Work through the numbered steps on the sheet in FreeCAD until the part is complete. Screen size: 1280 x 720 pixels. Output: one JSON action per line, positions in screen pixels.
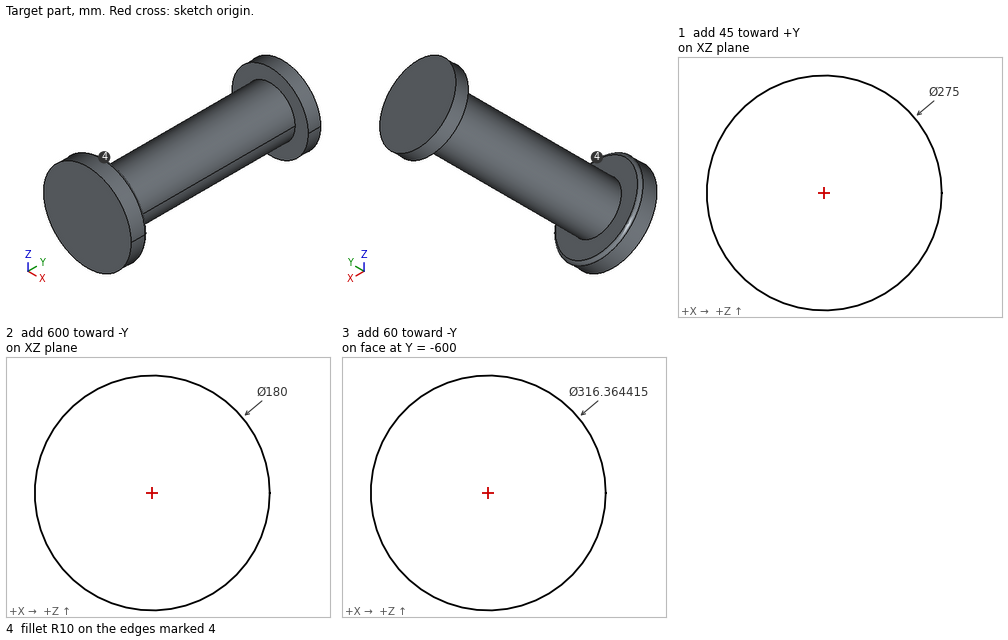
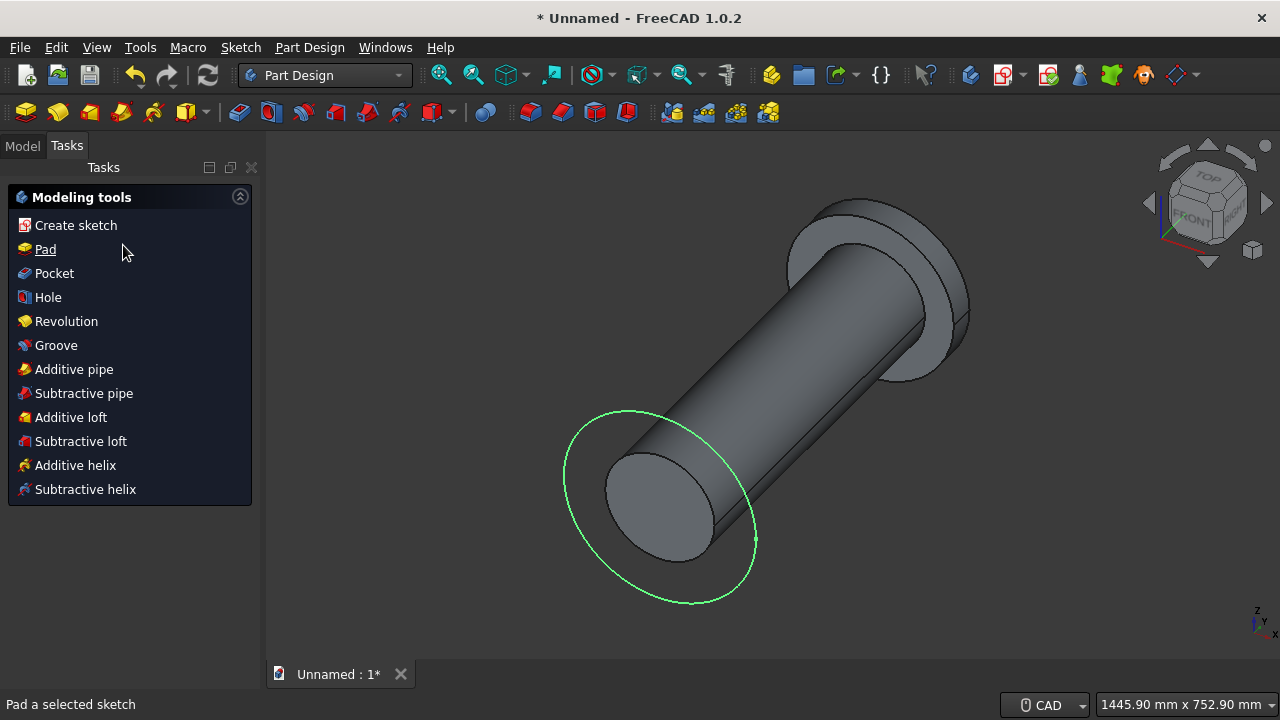
{"action": "left_click", "coordinate": [26, 112]}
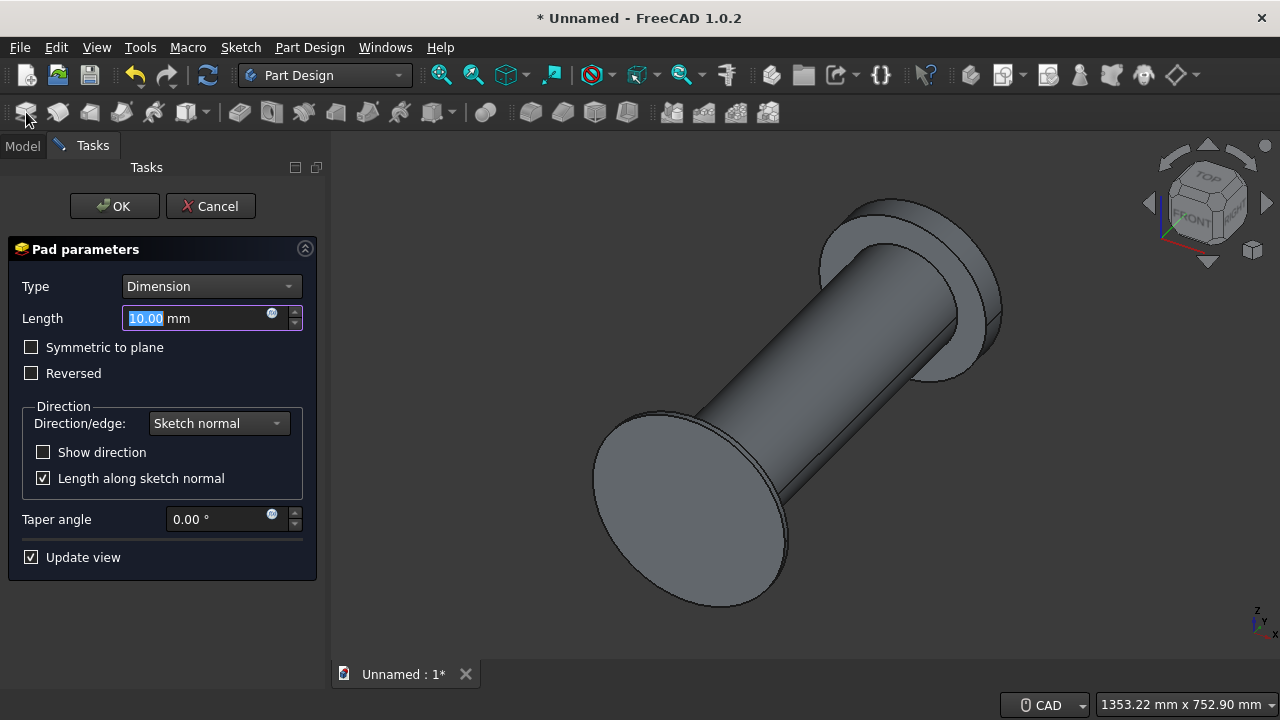
{"action": "type", "text": "60"}
{"action": "key", "text": "Tab"}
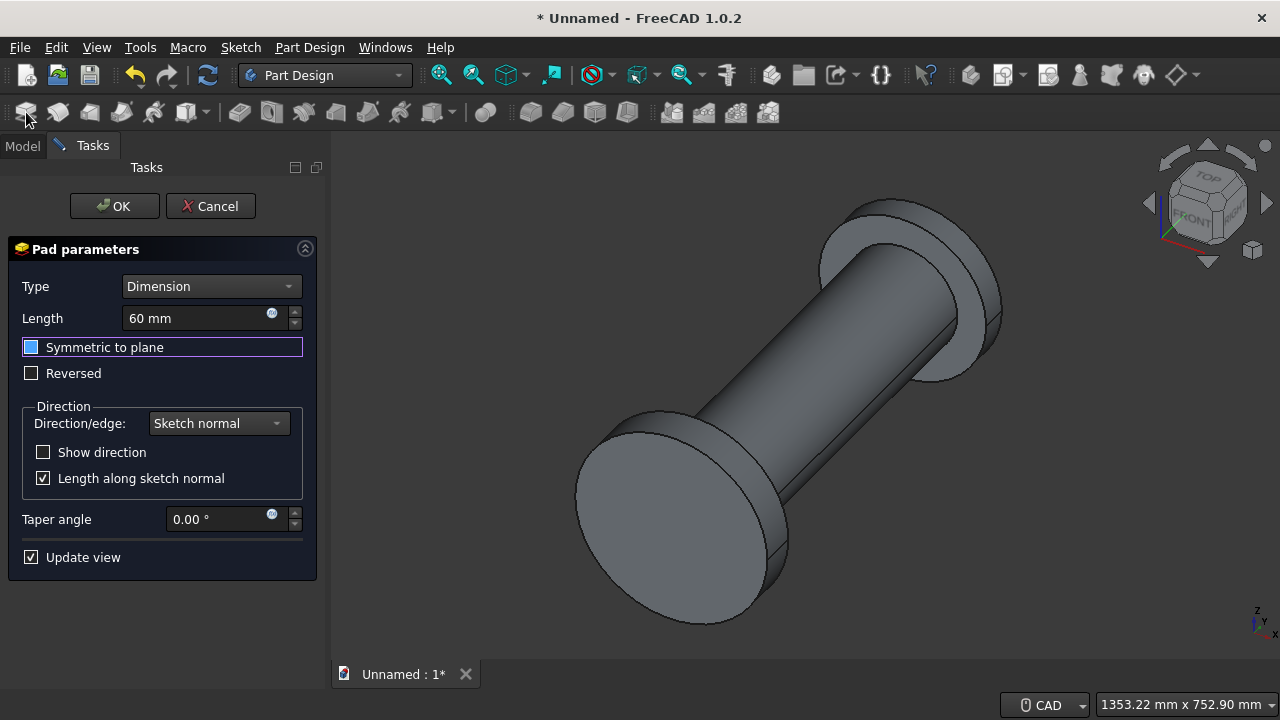
{"action": "left_click", "coordinate": [115, 206]}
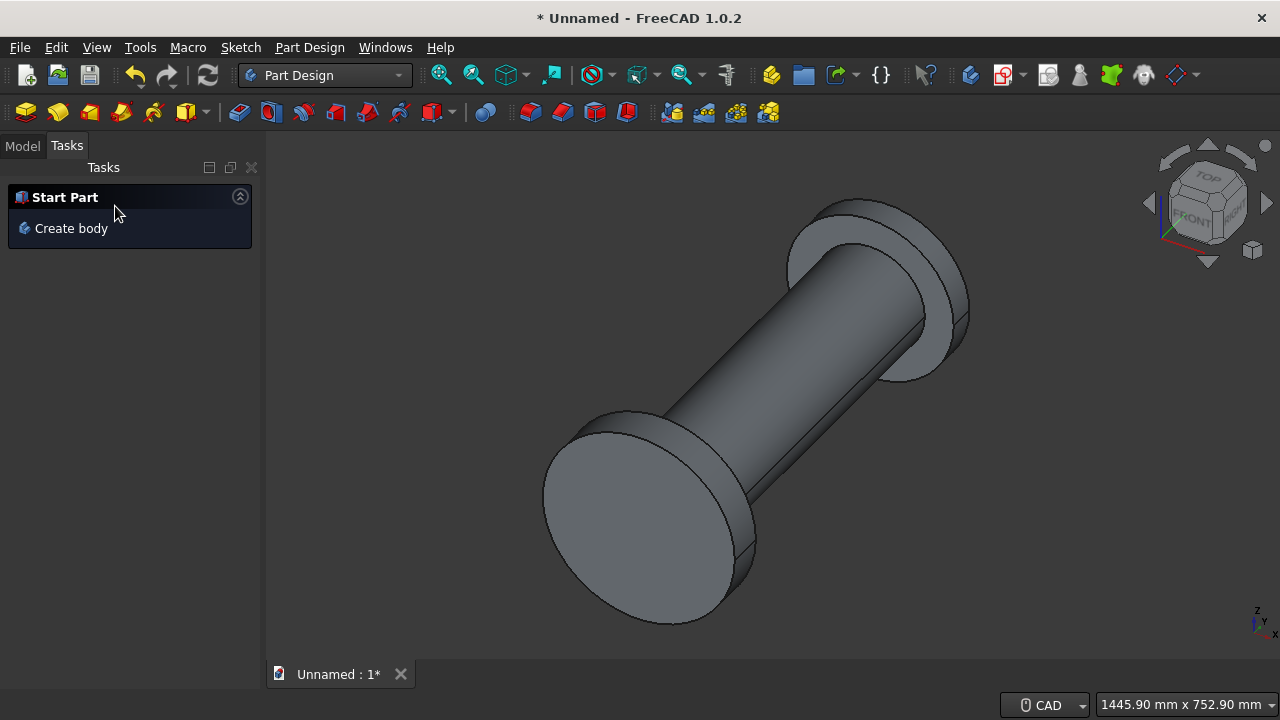
{"action": "key", "text": "0"}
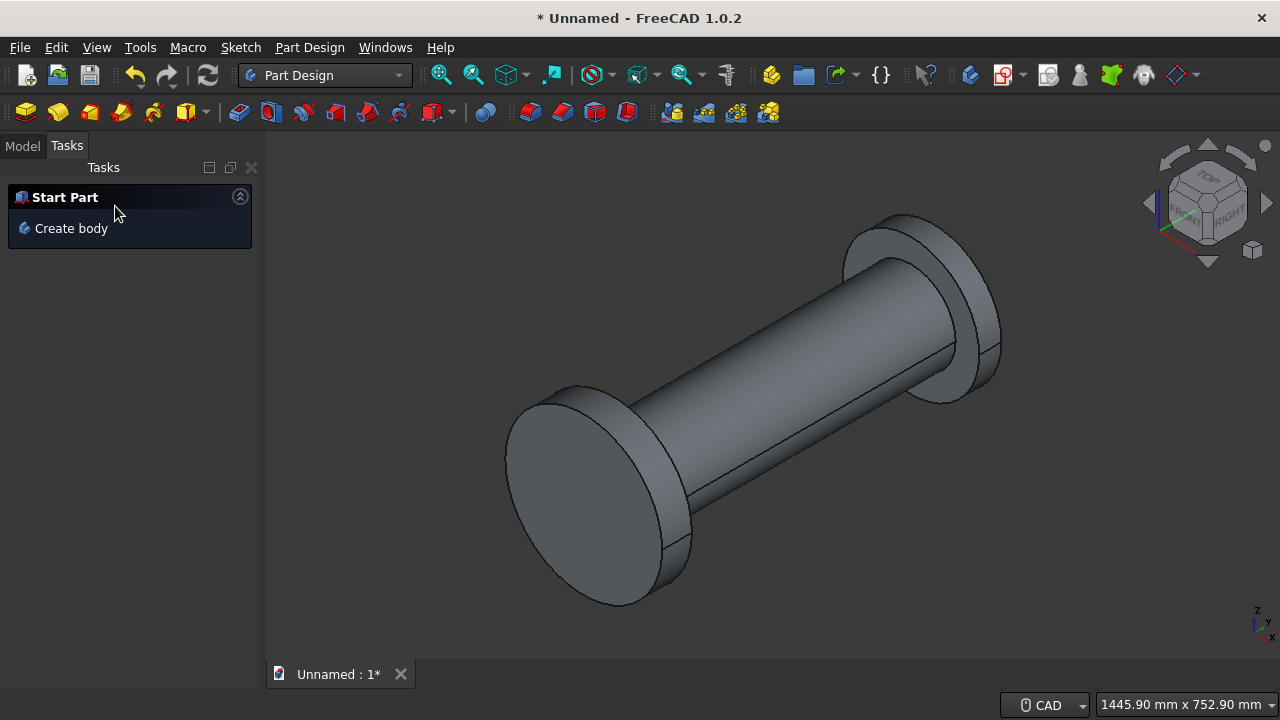
{"action": "key", "text": "2"}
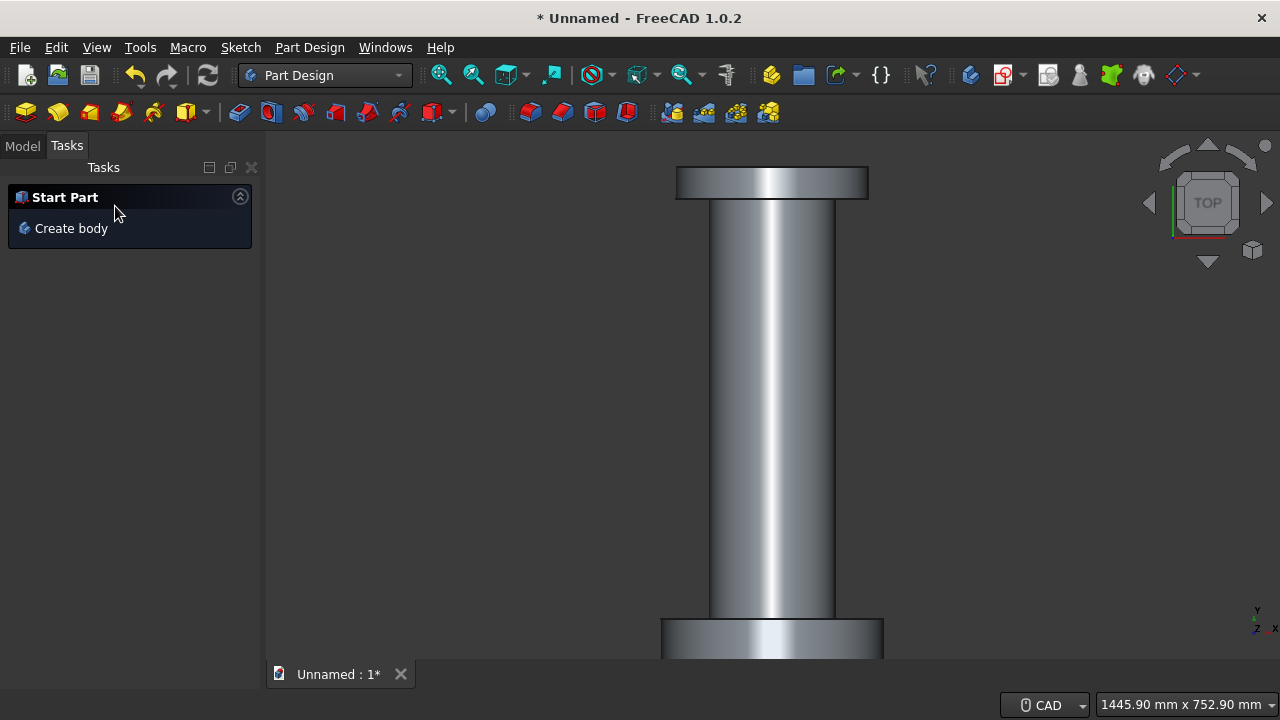
{"action": "key", "text": "v f"}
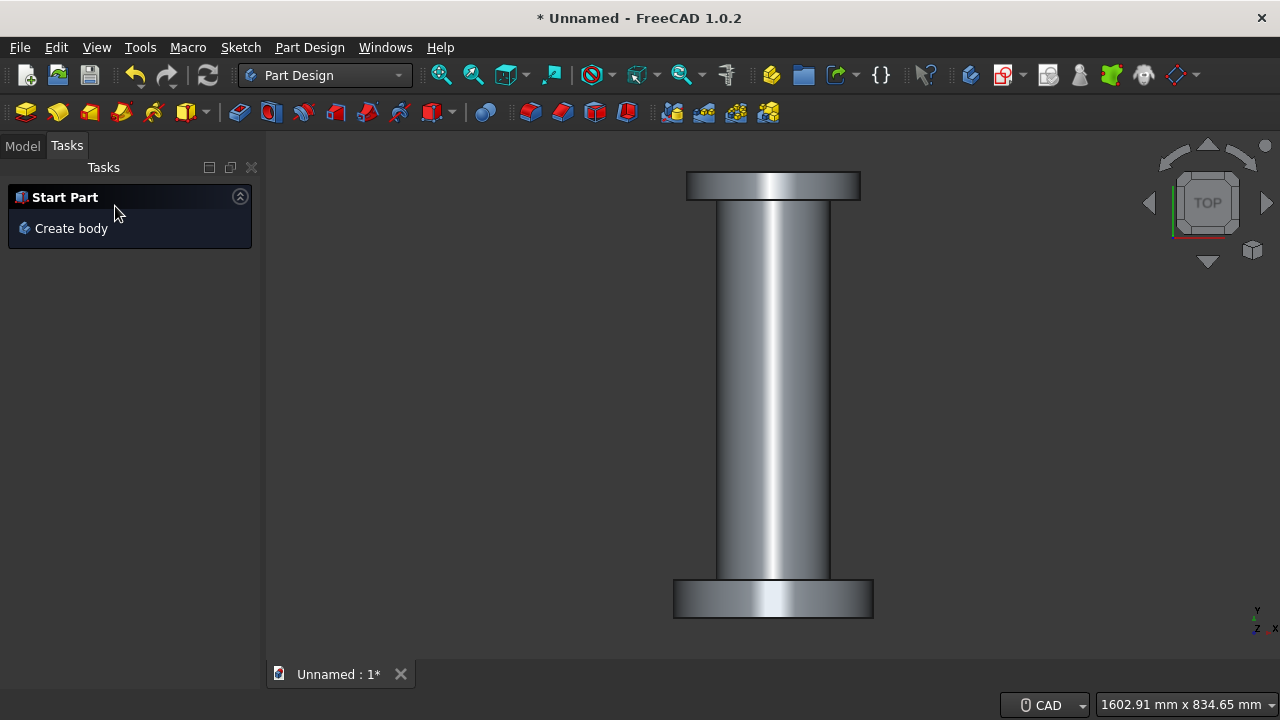
{"action": "left_click", "coordinate": [692, 579]}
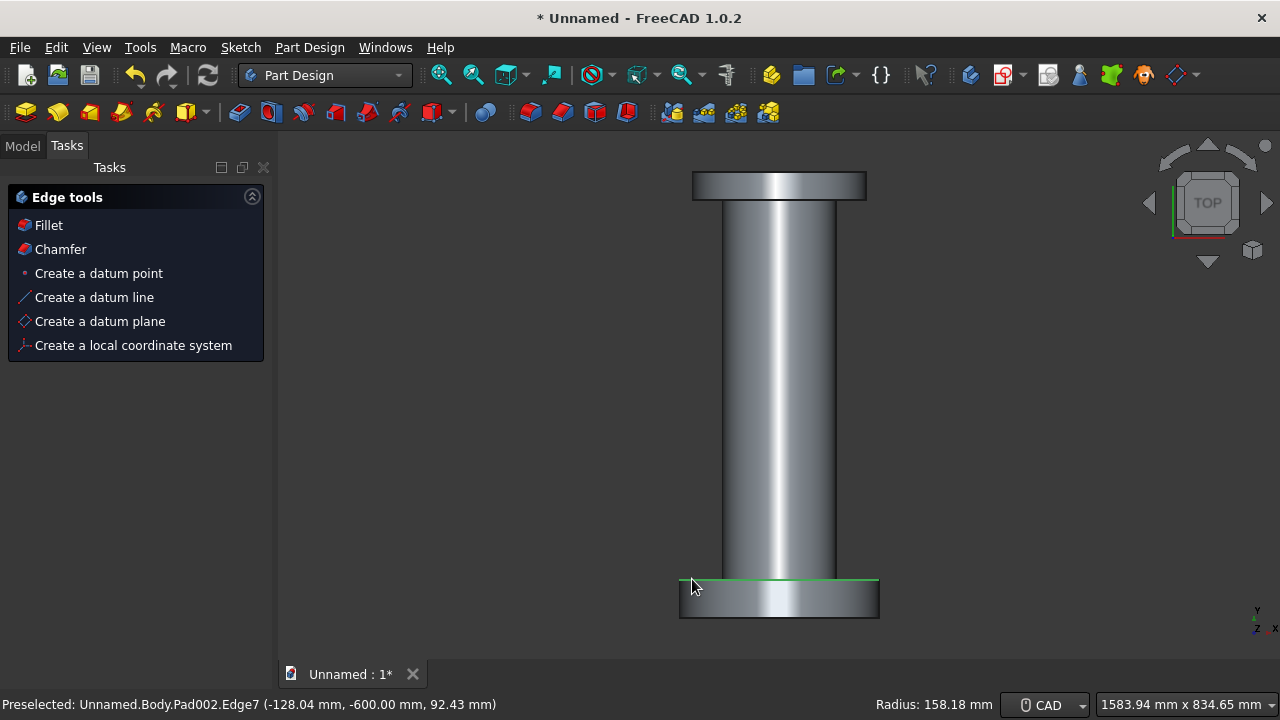
{"action": "left_click", "coordinate": [532, 112]}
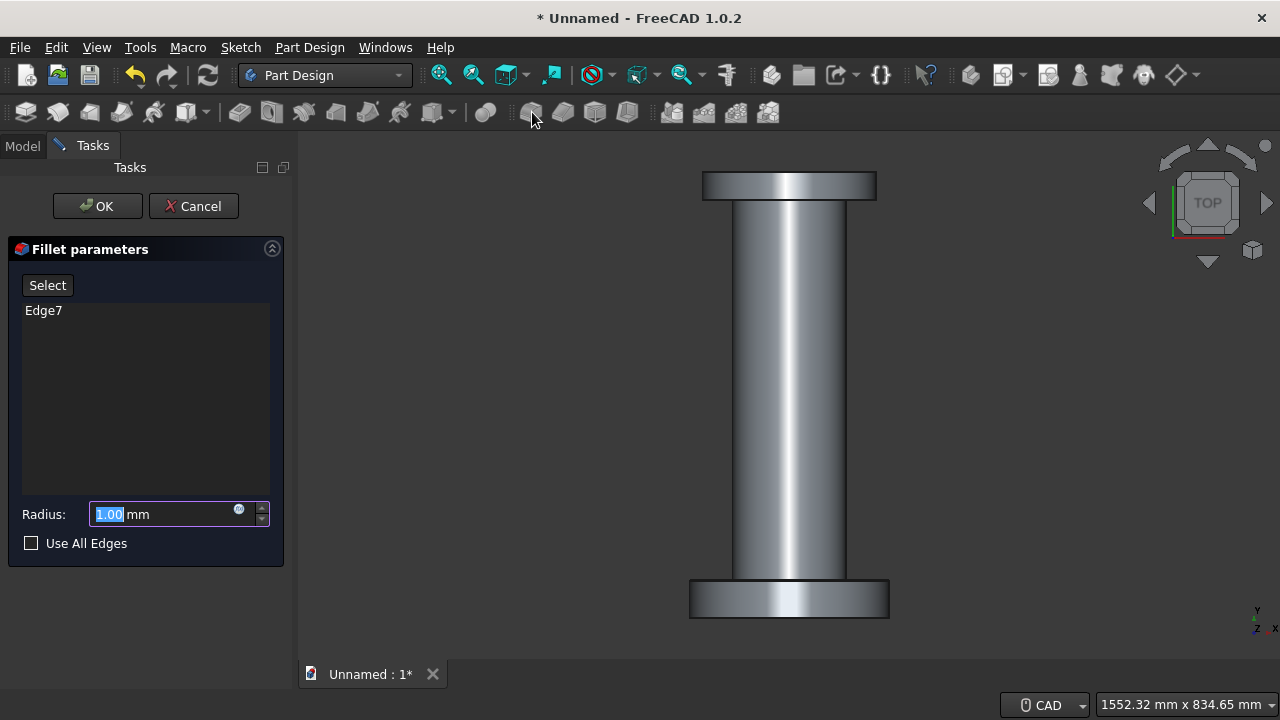
{"action": "type", "text": "10"}
{"action": "key", "text": "Tab"}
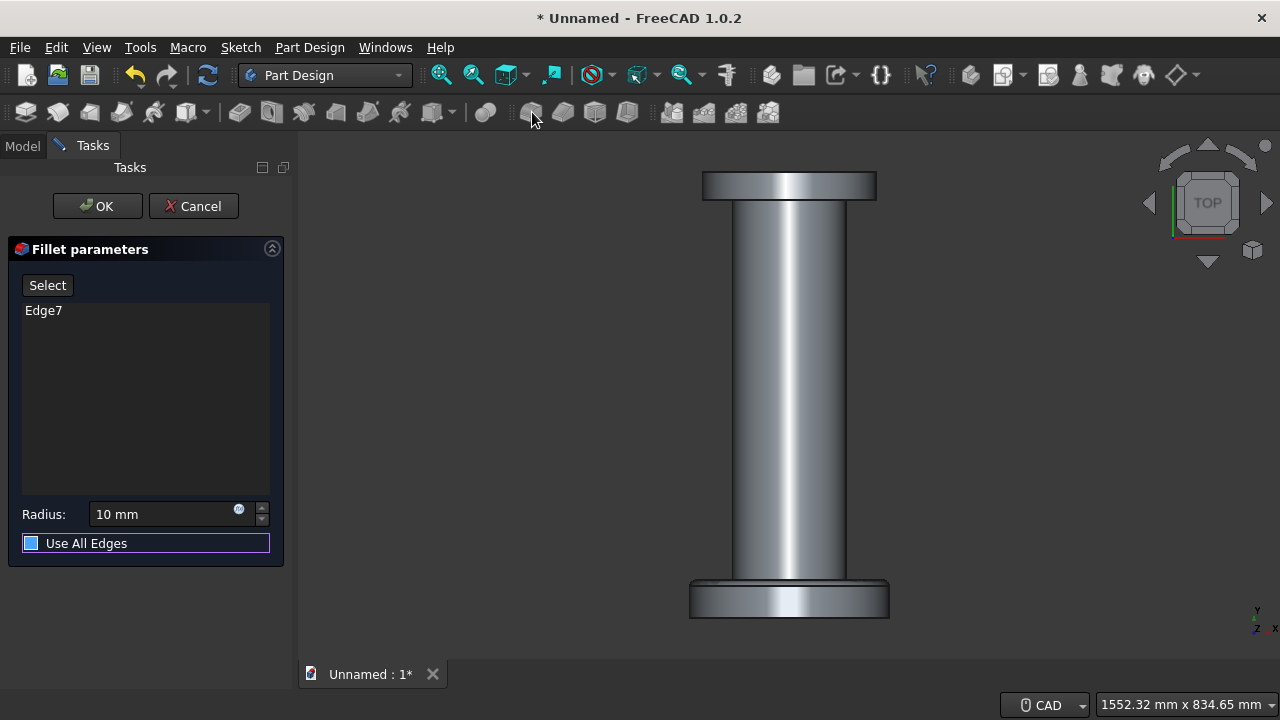
{"action": "left_click", "coordinate": [98, 206]}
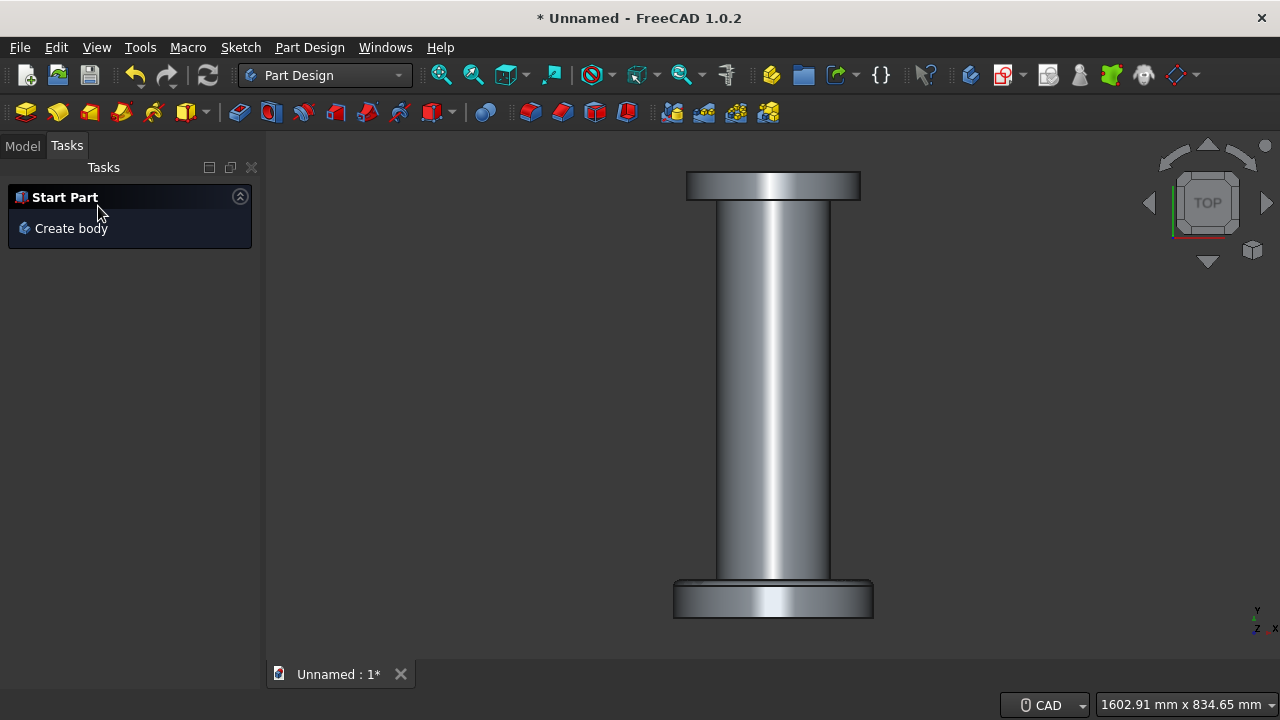
{"action": "key", "text": "0"}